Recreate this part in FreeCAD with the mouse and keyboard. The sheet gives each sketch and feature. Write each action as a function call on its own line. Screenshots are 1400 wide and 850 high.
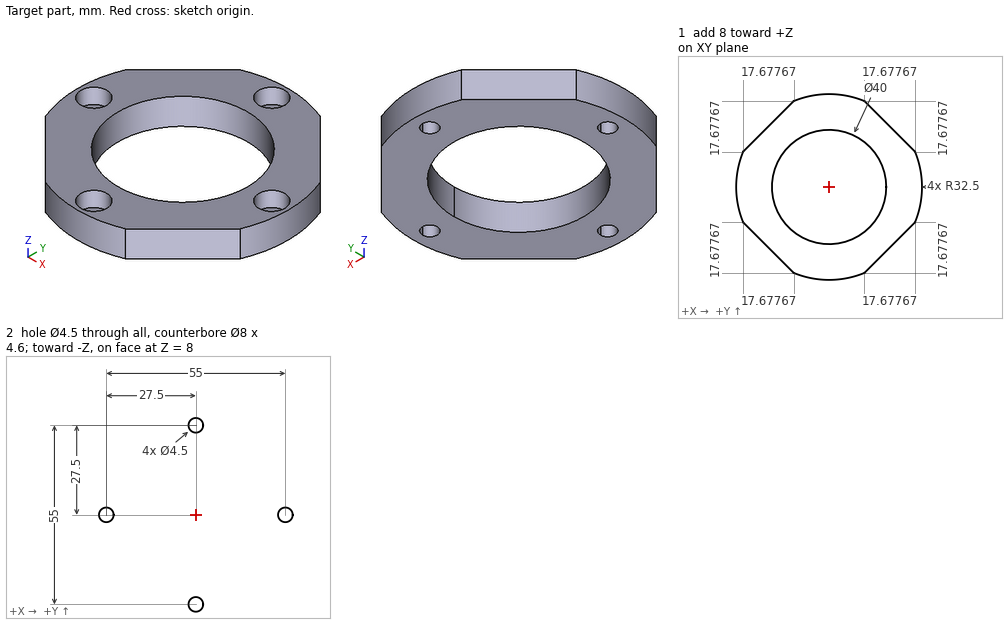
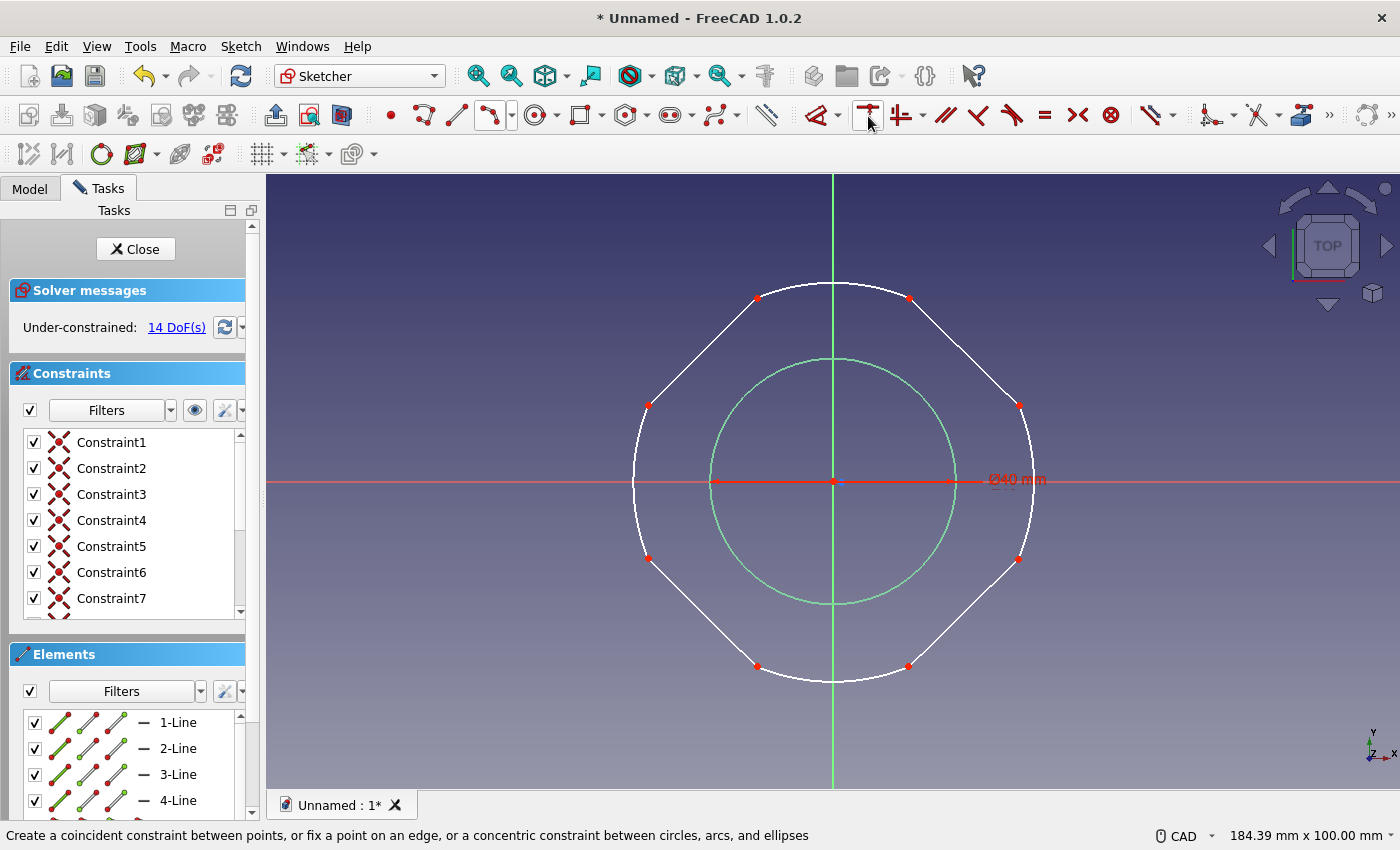
click(920, 394)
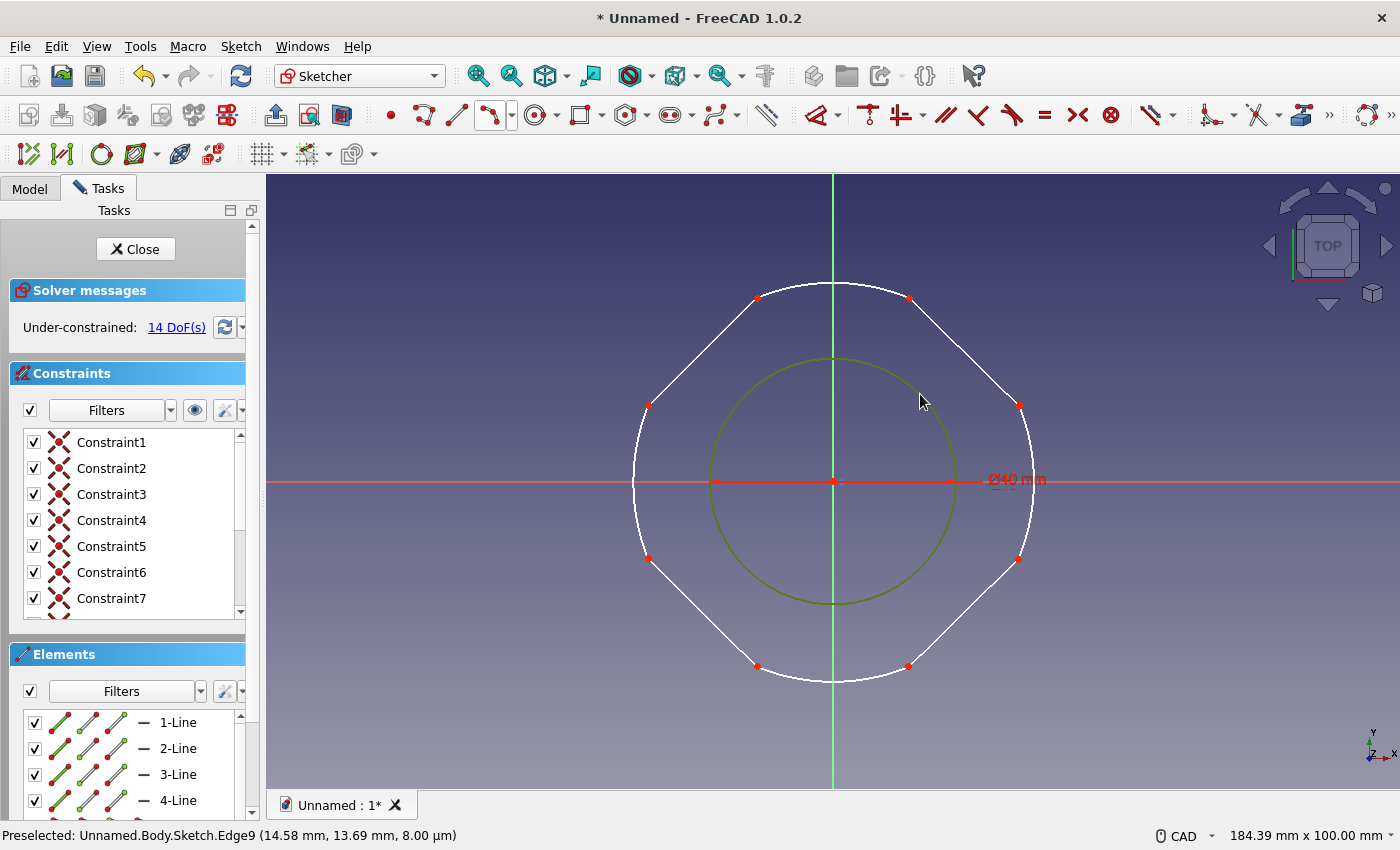
click(636, 451)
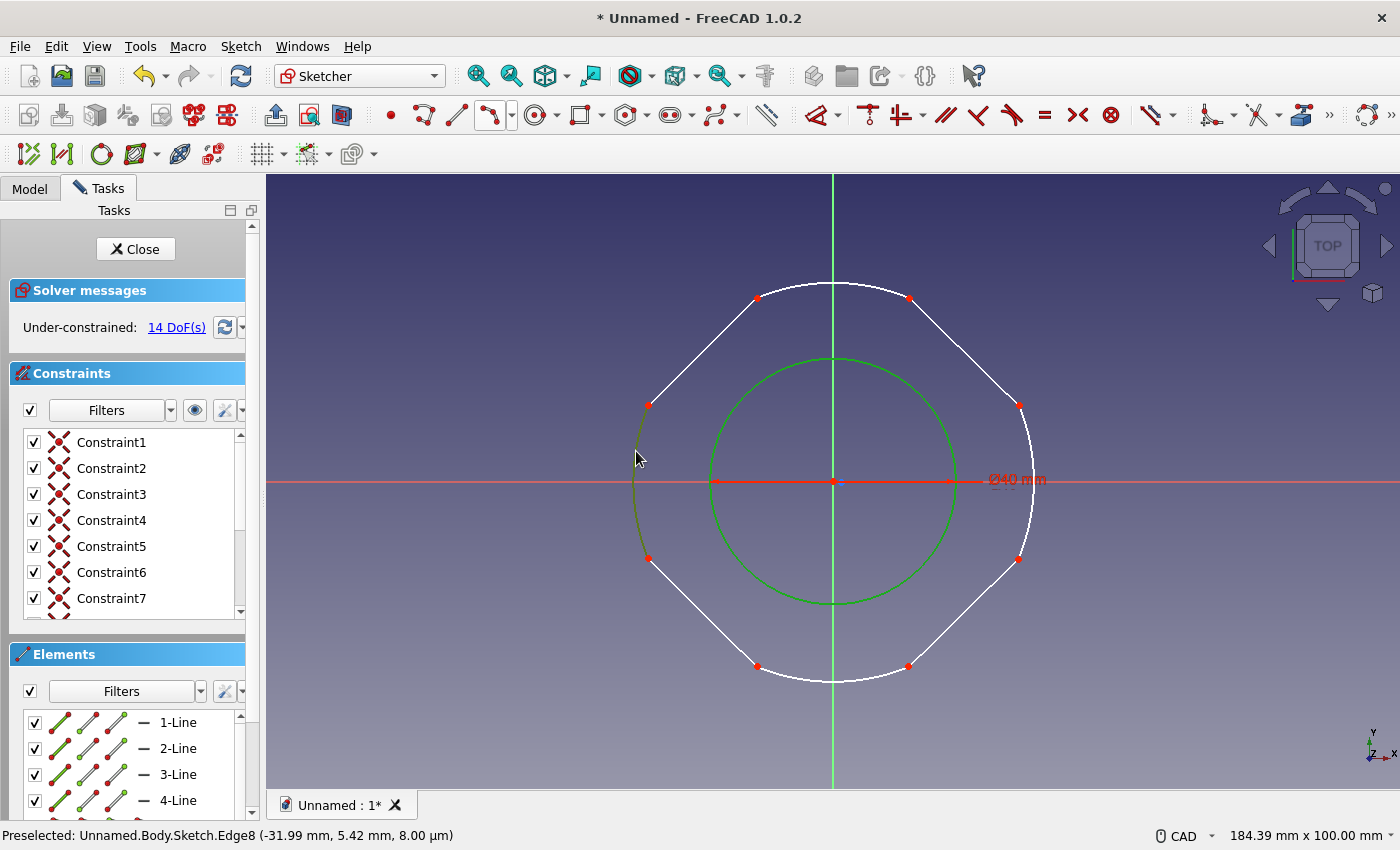
click(868, 116)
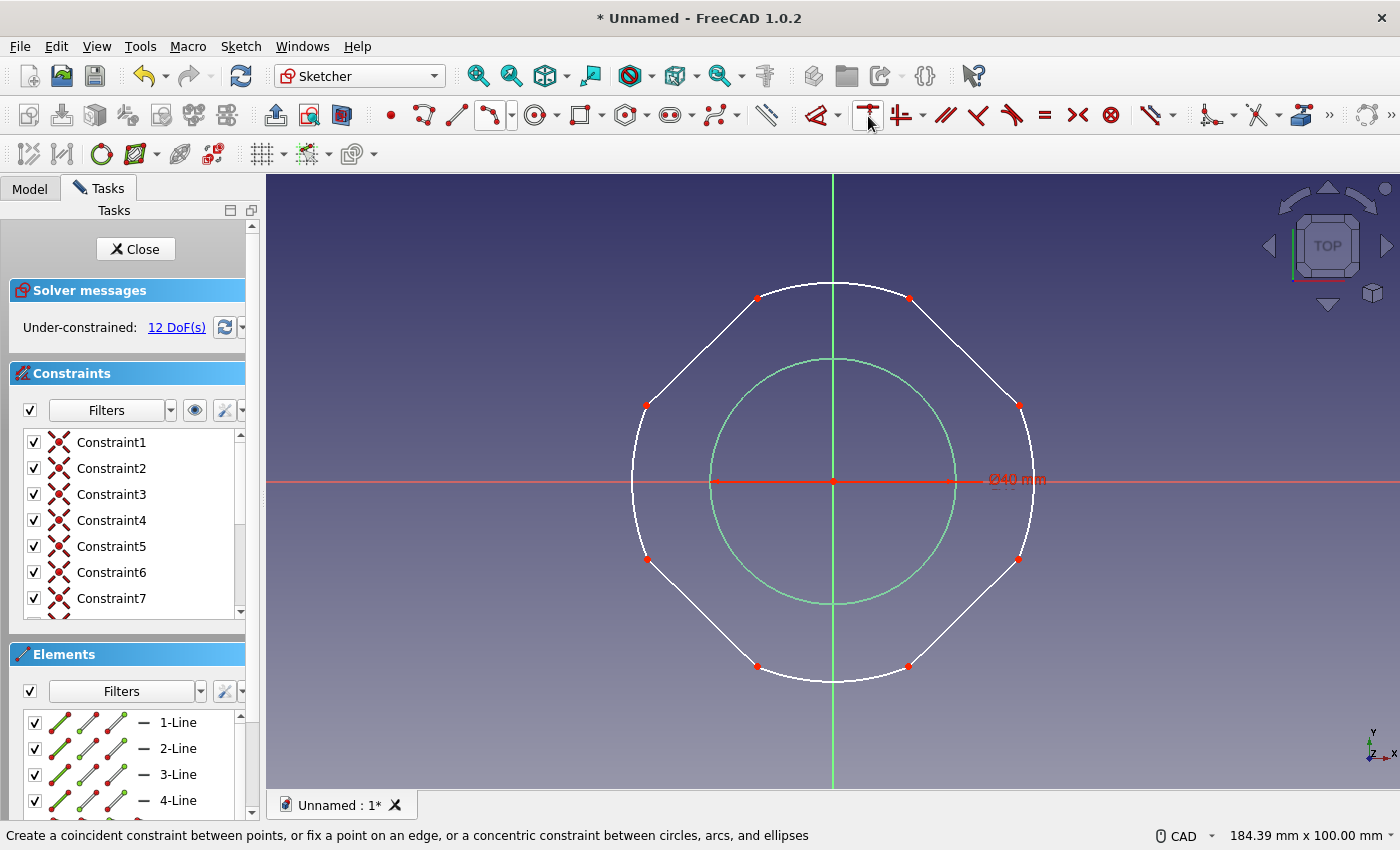
click(802, 679)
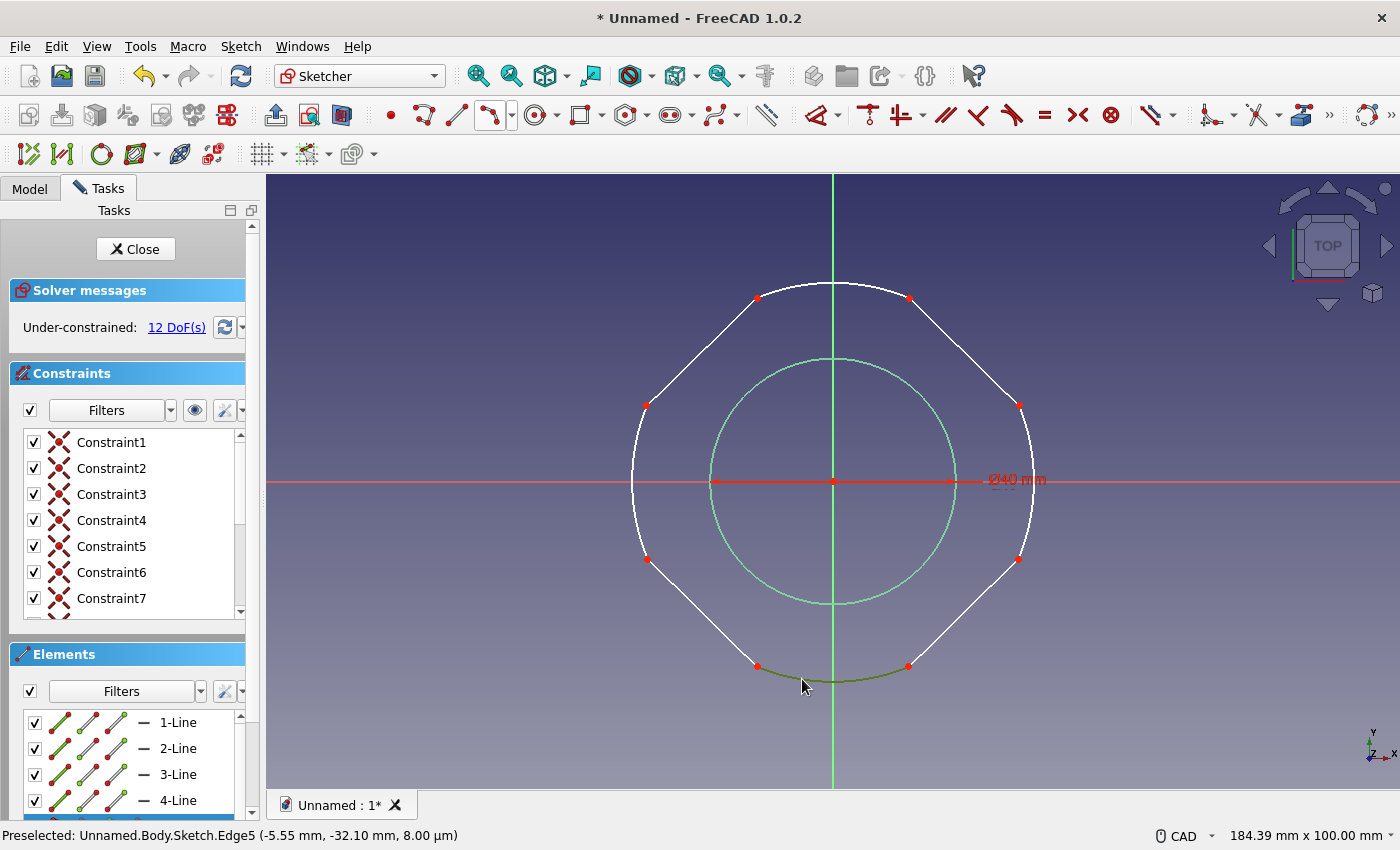
click(1031, 514)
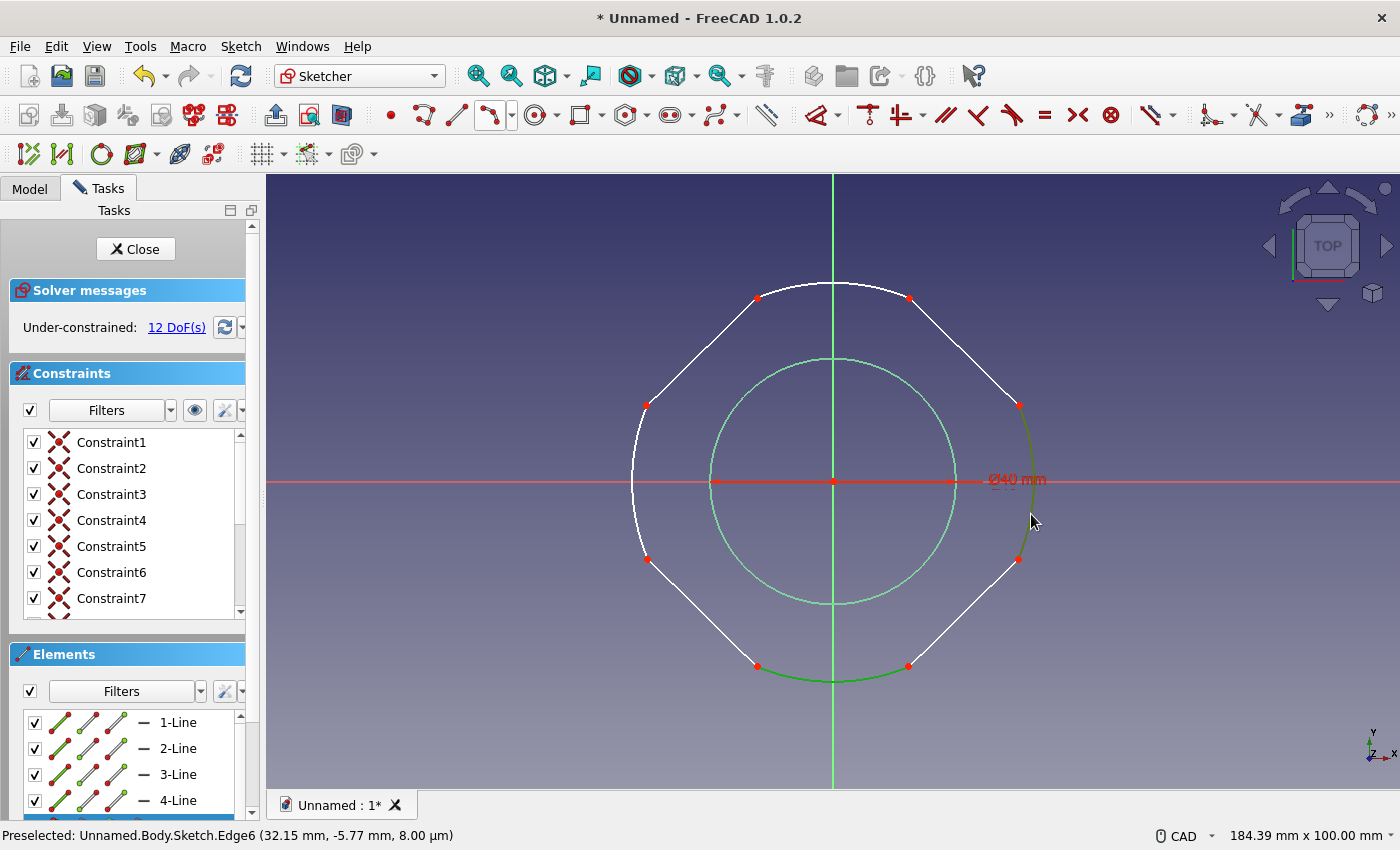
click(864, 285)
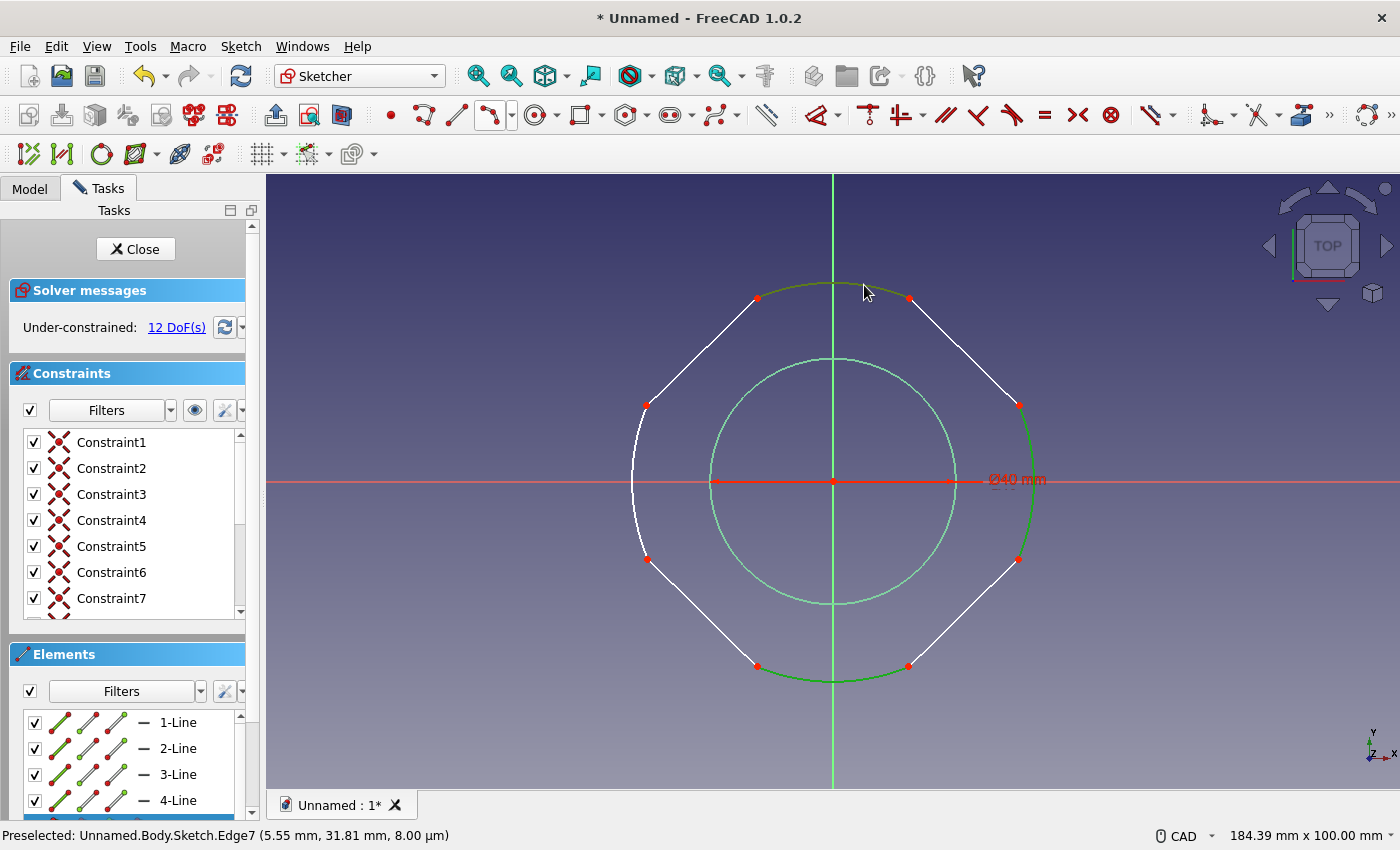
click(634, 451)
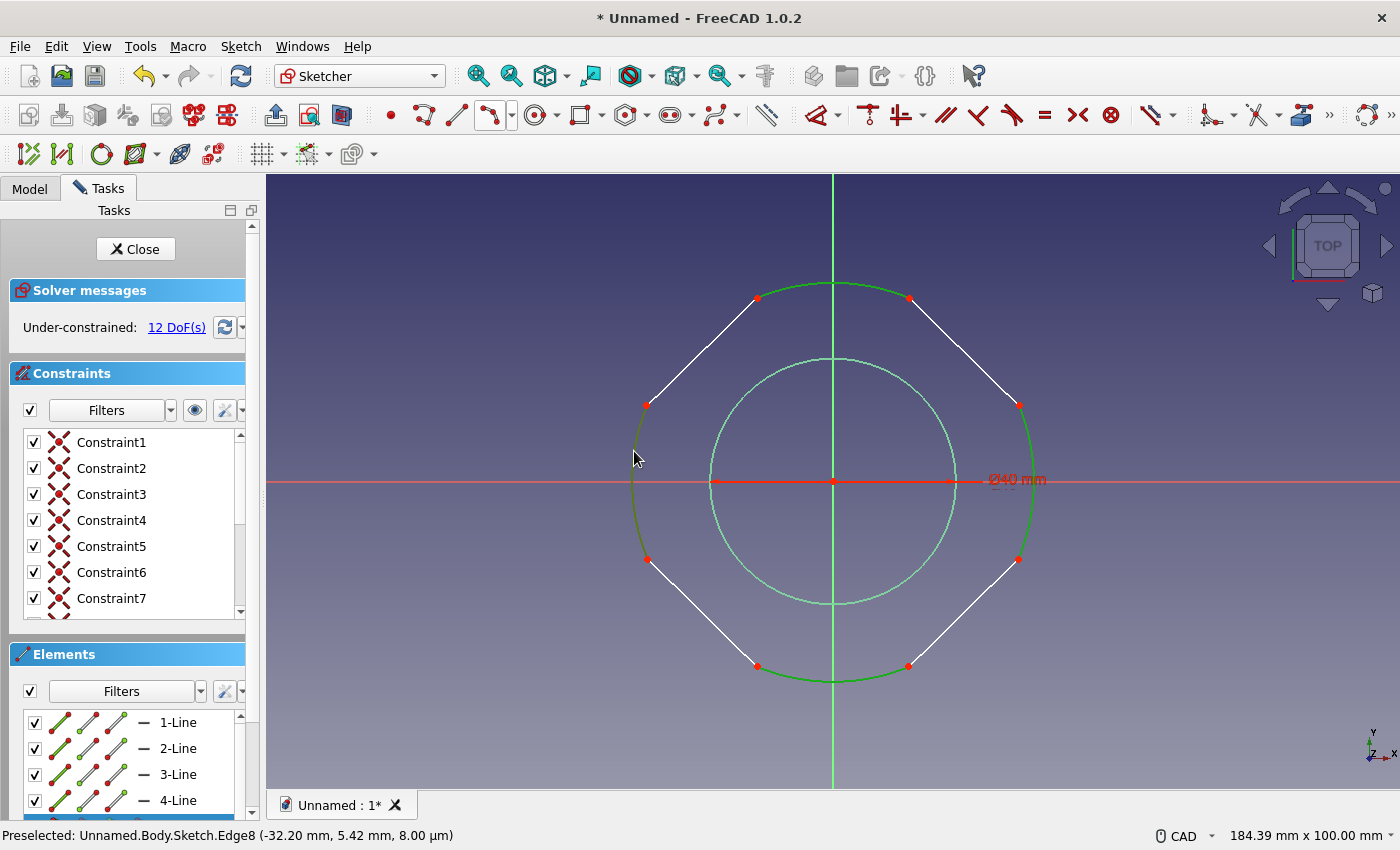
click(1045, 116)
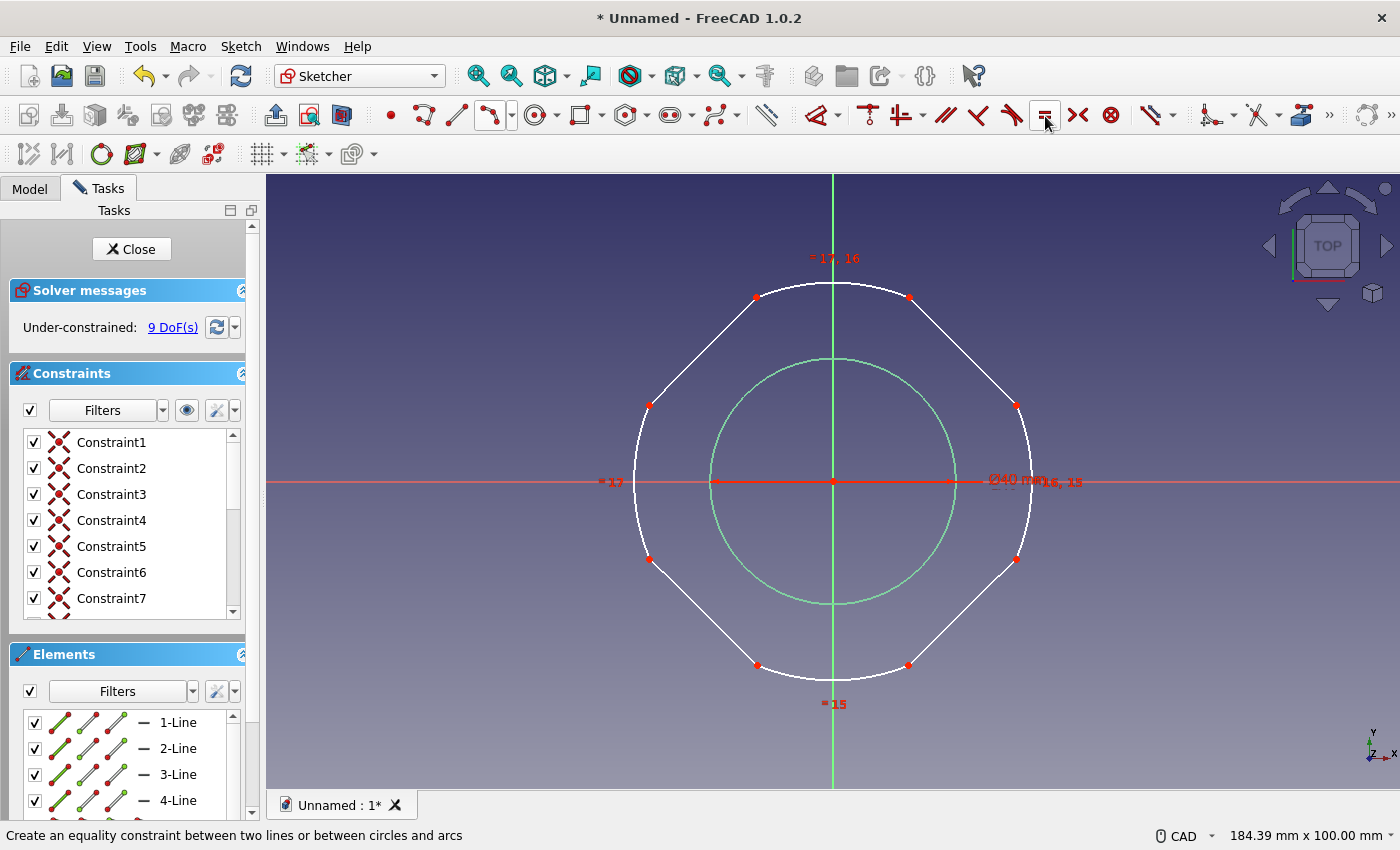
click(816, 116)